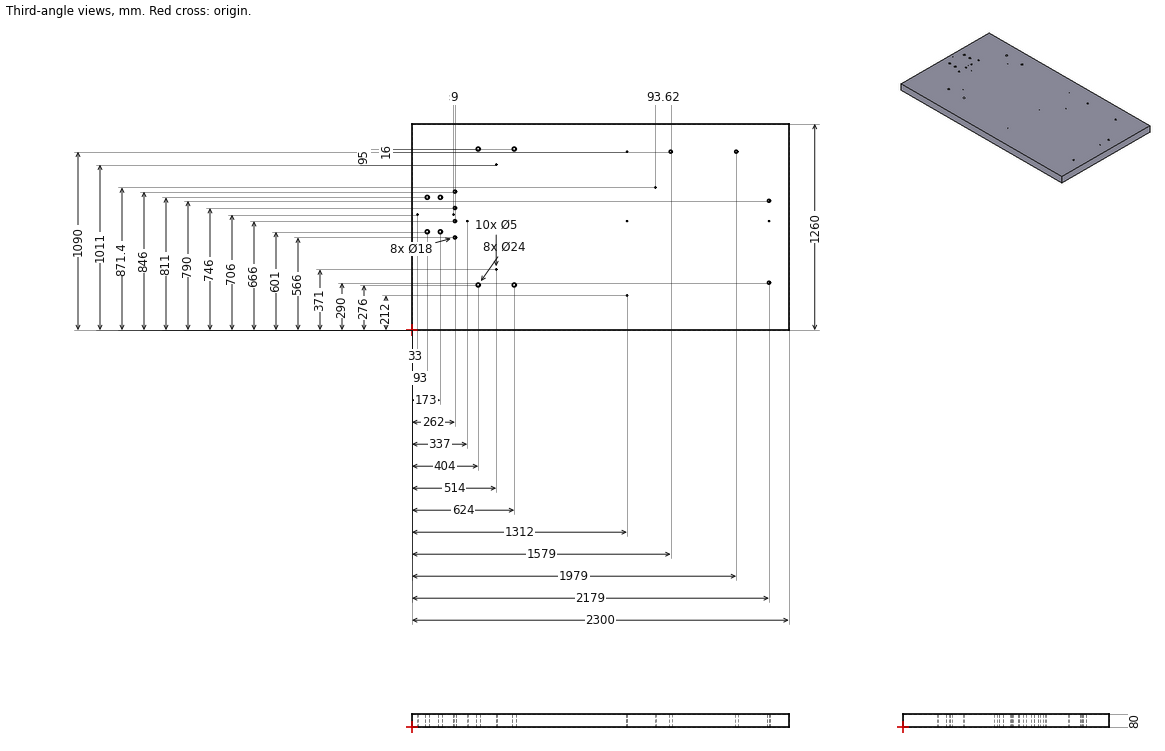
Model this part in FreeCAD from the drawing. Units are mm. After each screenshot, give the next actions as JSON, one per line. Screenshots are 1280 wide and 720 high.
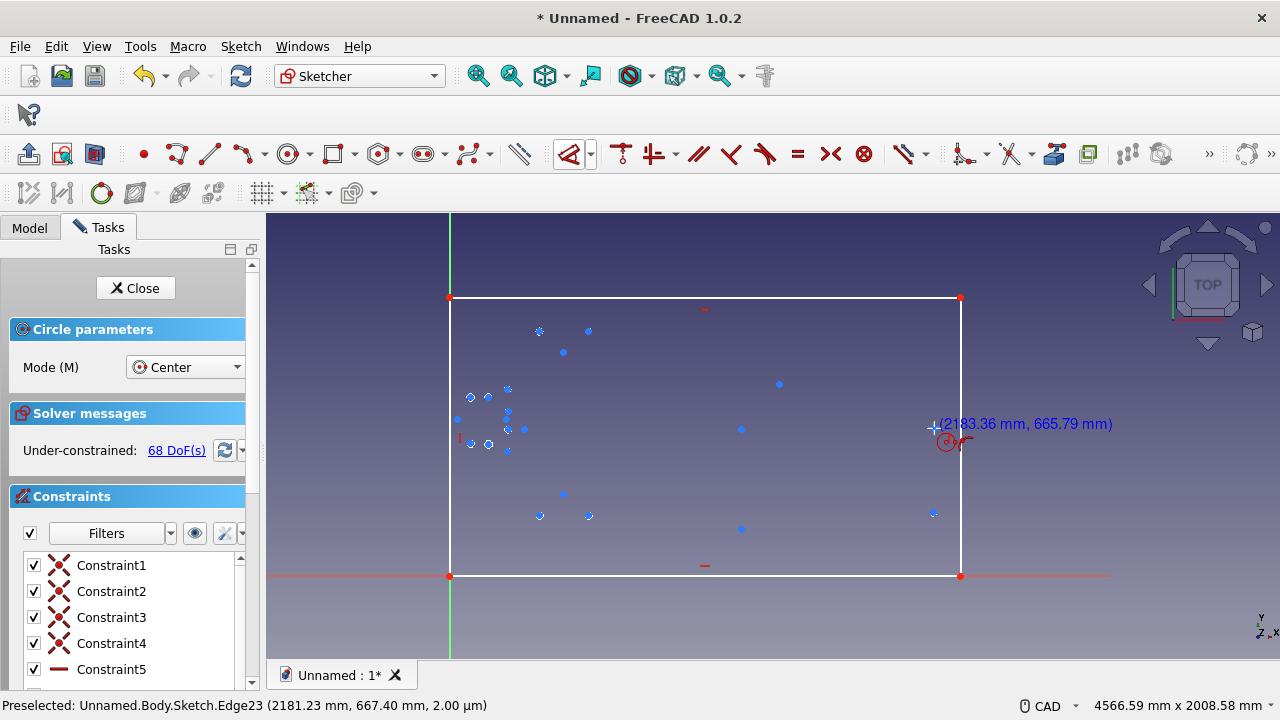
{"action": "scroll", "coordinate": [934, 401], "scroll_direction": "up", "scroll_amount": 13}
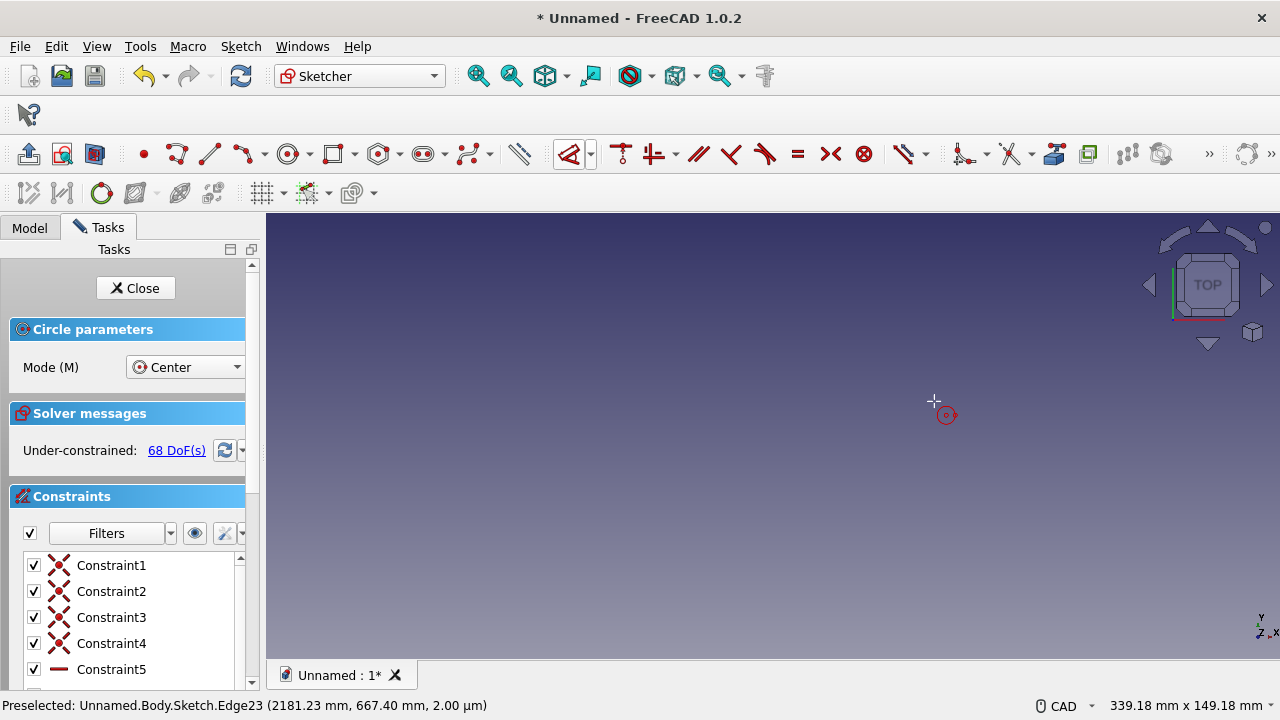
{"action": "scroll", "coordinate": [934, 401], "scroll_direction": "down", "scroll_amount": 13}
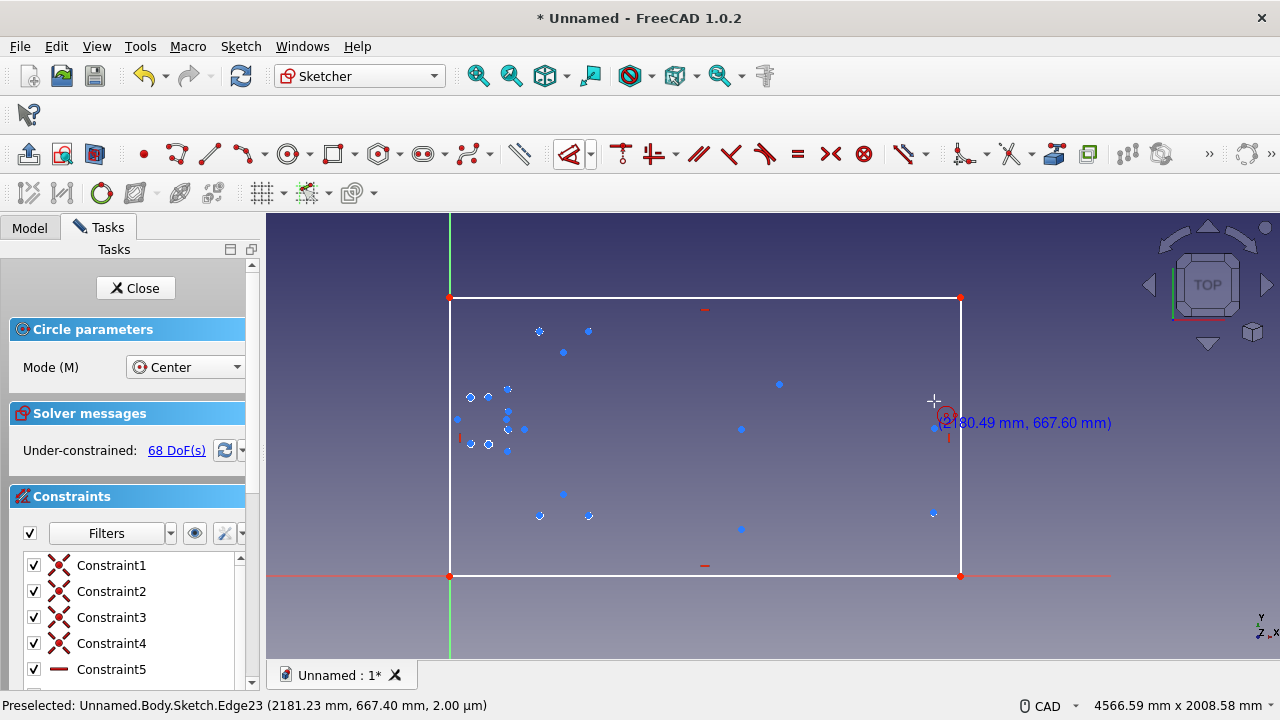
{"action": "left_click", "coordinate": [934, 401]}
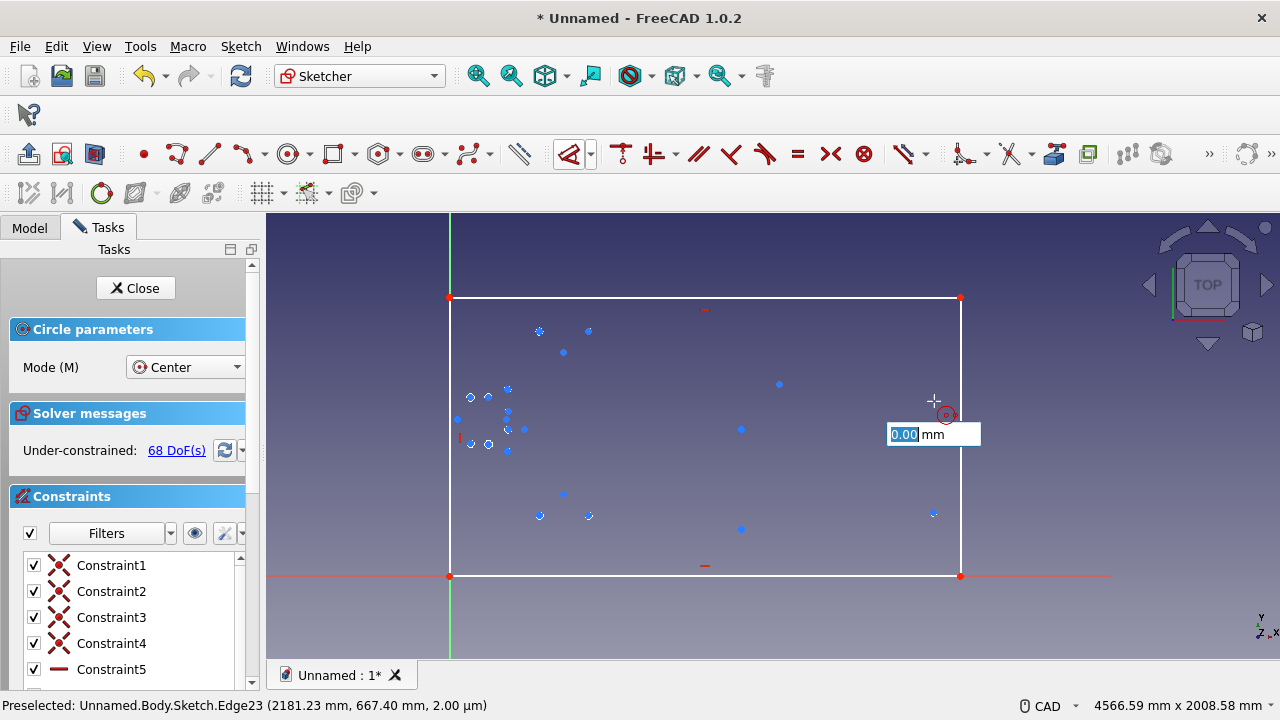
{"action": "scroll", "coordinate": [935, 400], "scroll_direction": "up", "scroll_amount": 11}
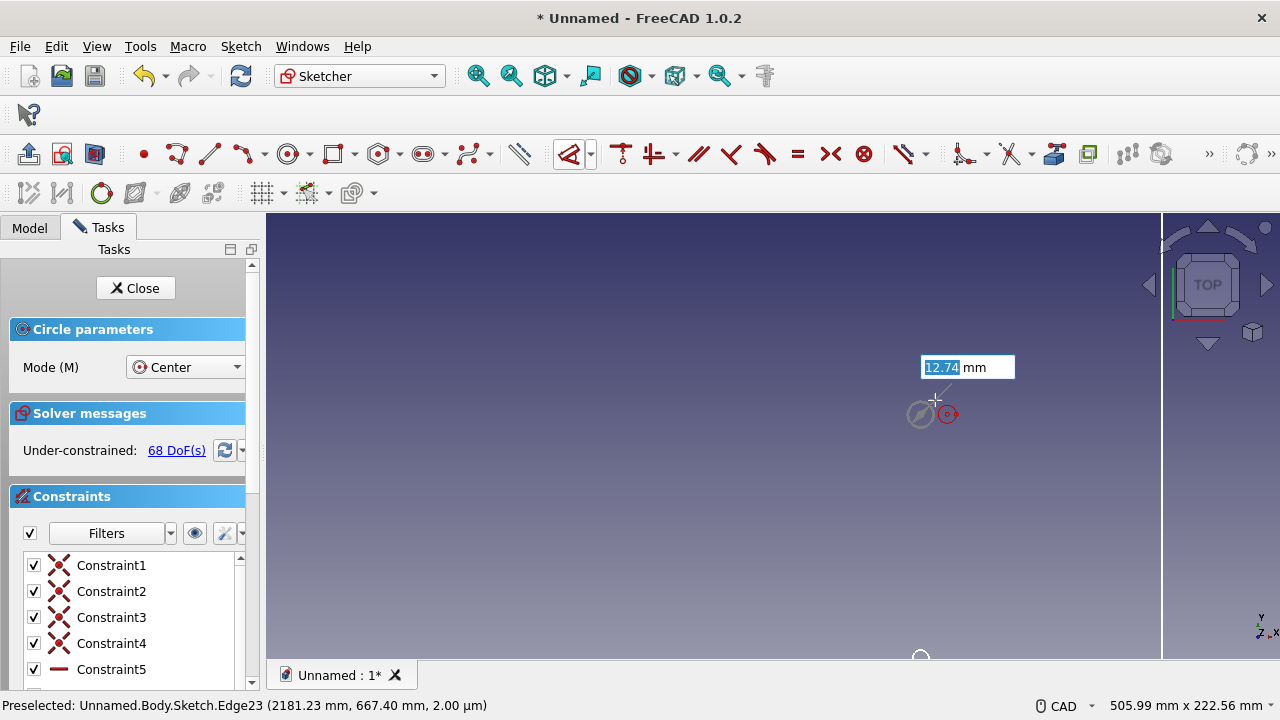
{"action": "left_click", "coordinate": [930, 392]}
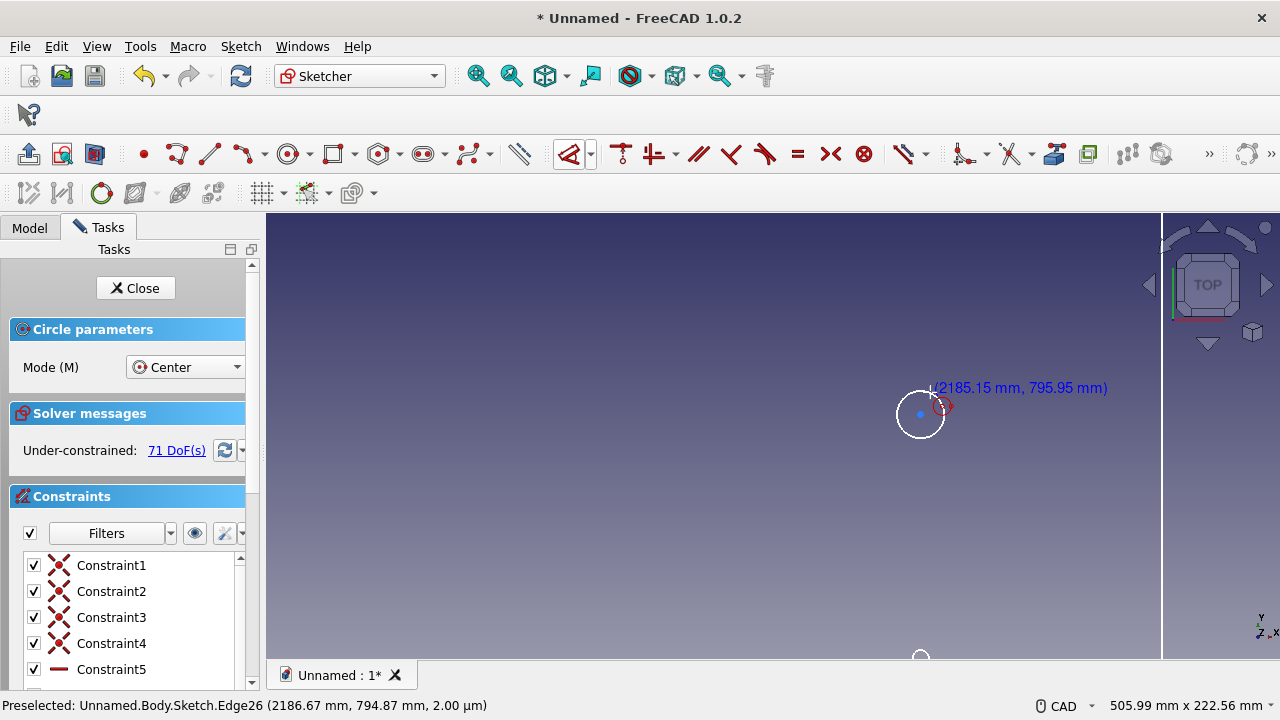
{"action": "scroll", "coordinate": [935, 400], "scroll_direction": "down", "scroll_amount": 11}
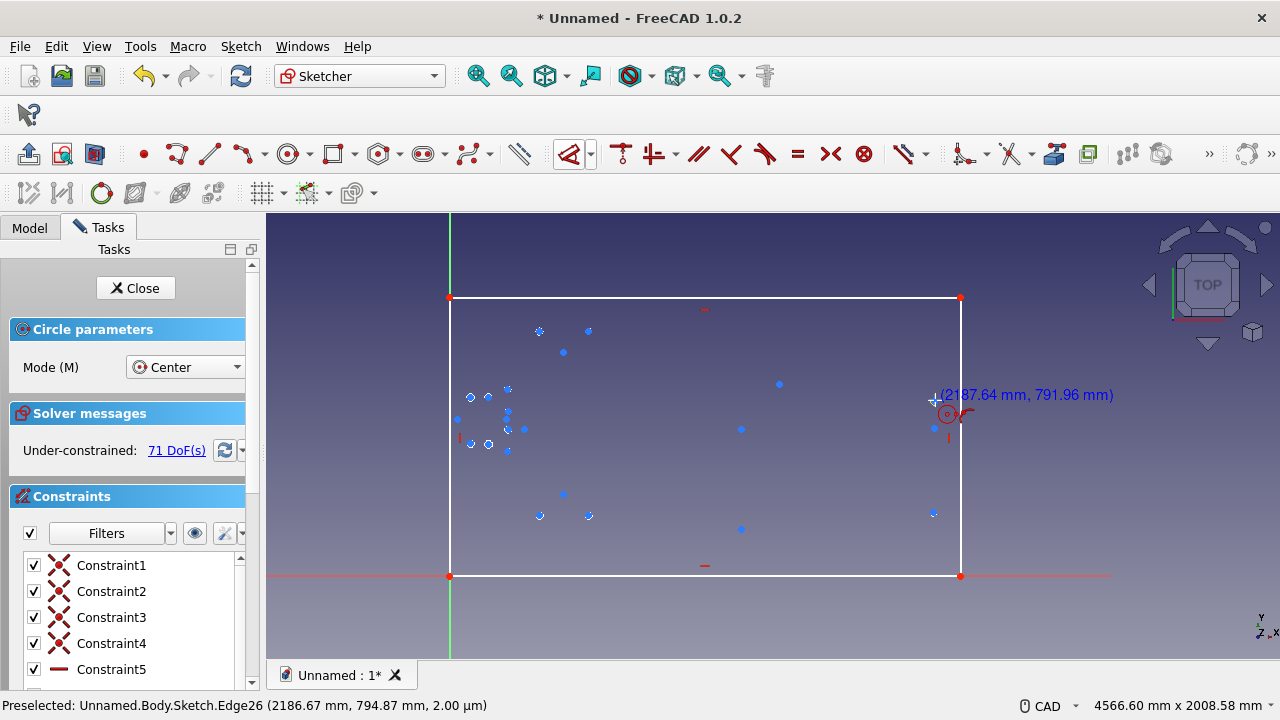
{"action": "scroll", "coordinate": [741, 334], "scroll_direction": "up", "scroll_amount": 19}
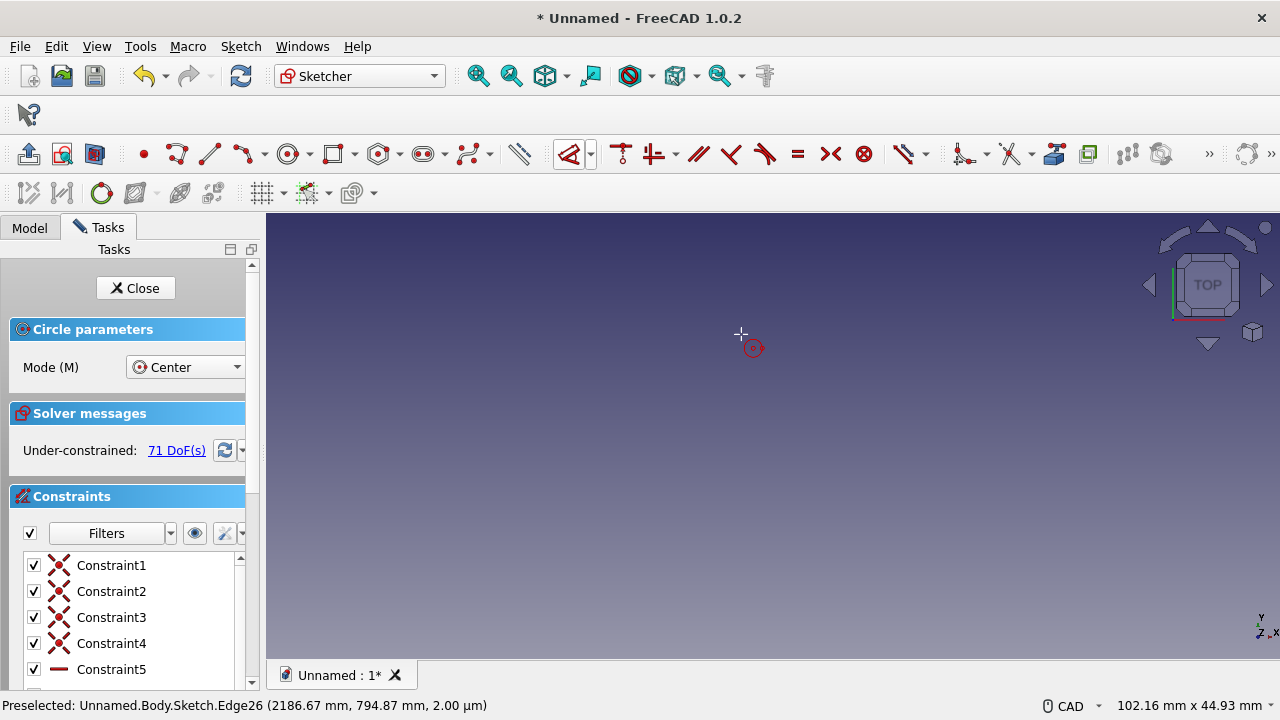
{"action": "scroll", "coordinate": [704, 436], "scroll_direction": "down", "scroll_amount": 15}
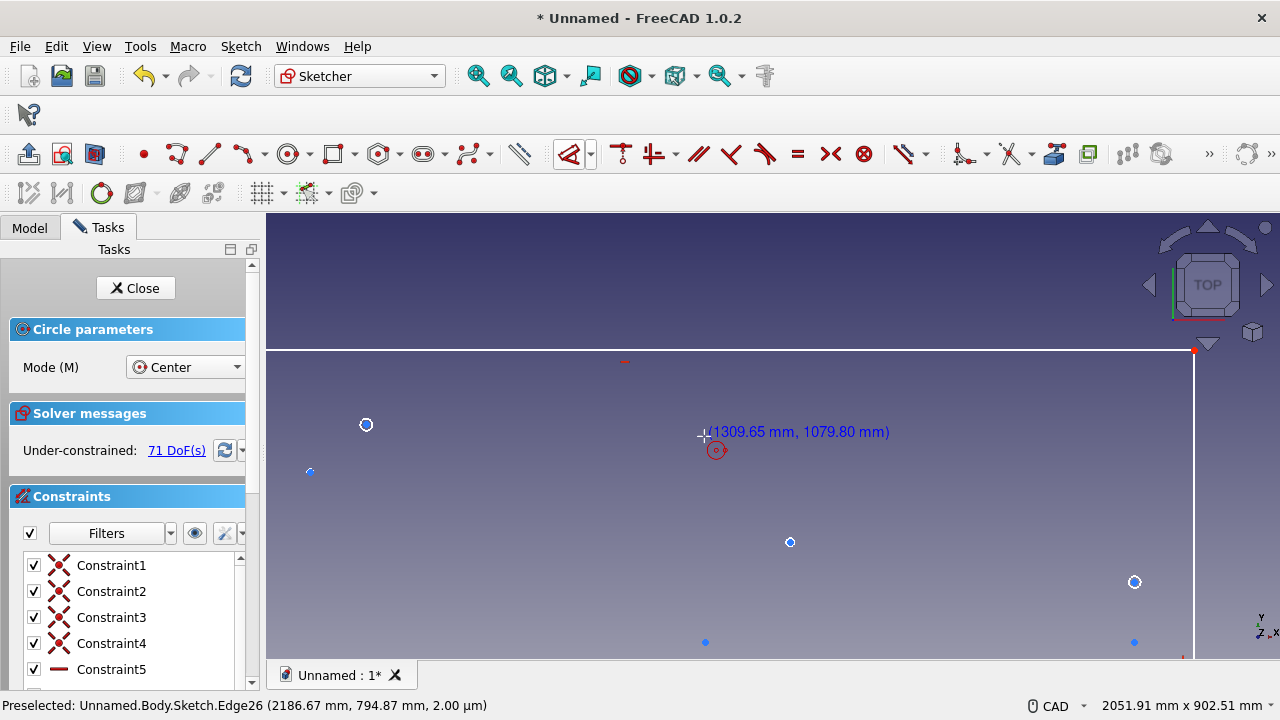
{"action": "scroll", "coordinate": [769, 254], "scroll_direction": "down", "scroll_amount": 4}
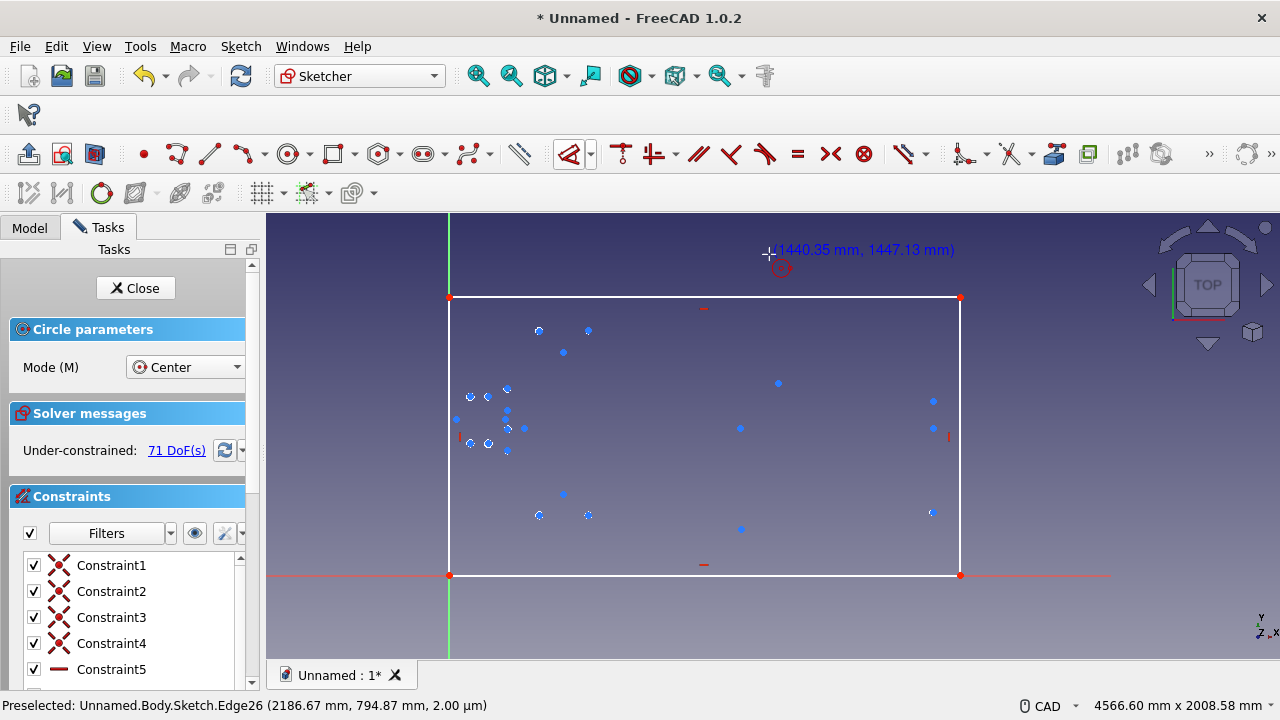
{"action": "left_click", "coordinate": [741, 334]}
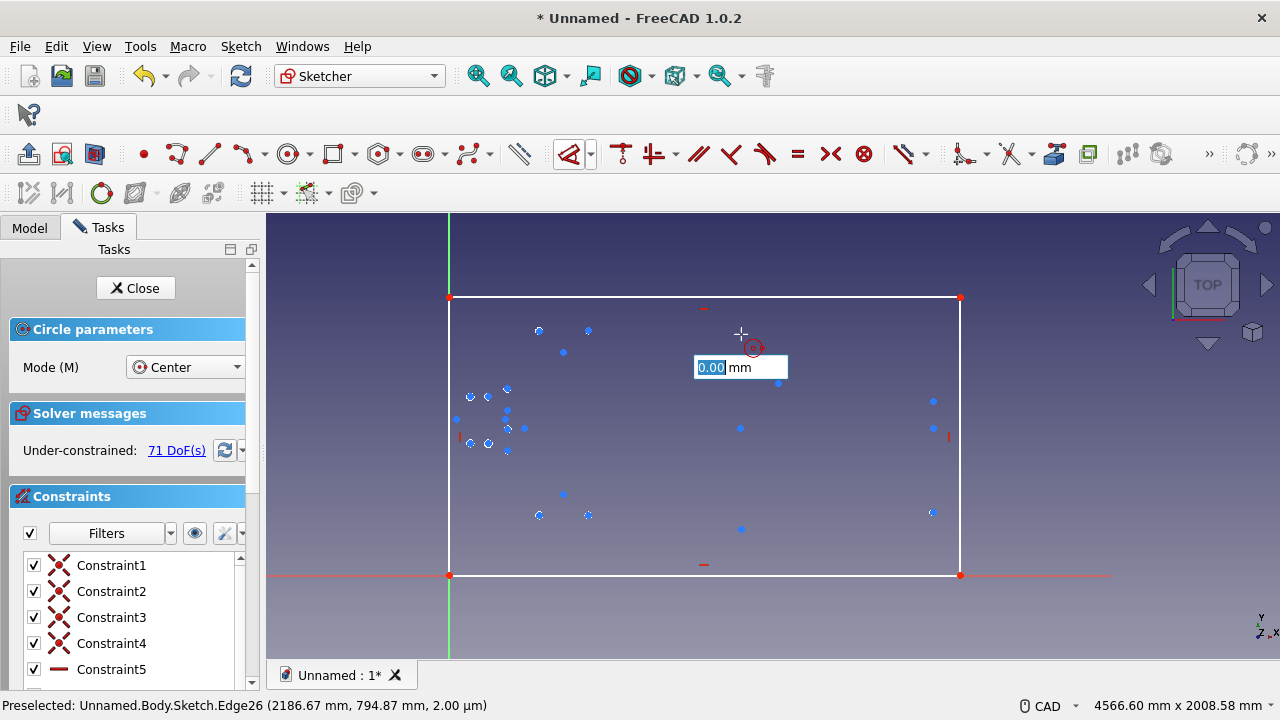
{"action": "scroll", "coordinate": [741, 333], "scroll_direction": "up", "scroll_amount": 17}